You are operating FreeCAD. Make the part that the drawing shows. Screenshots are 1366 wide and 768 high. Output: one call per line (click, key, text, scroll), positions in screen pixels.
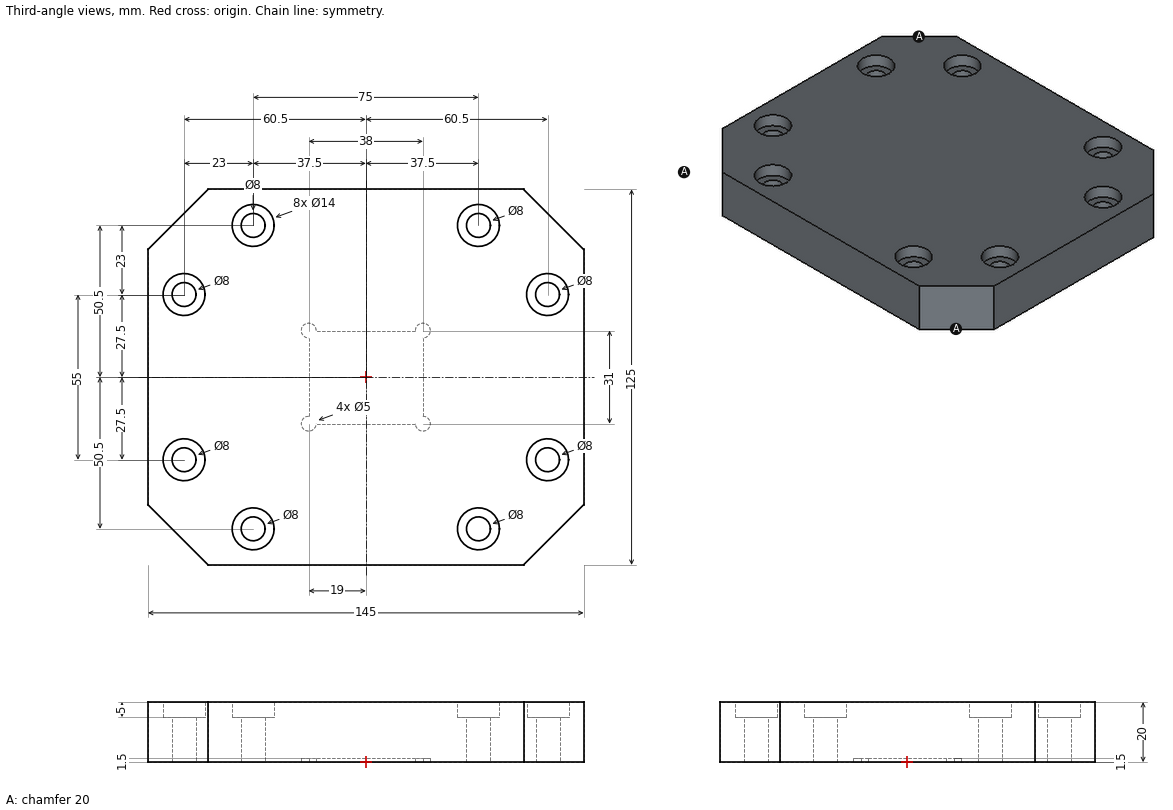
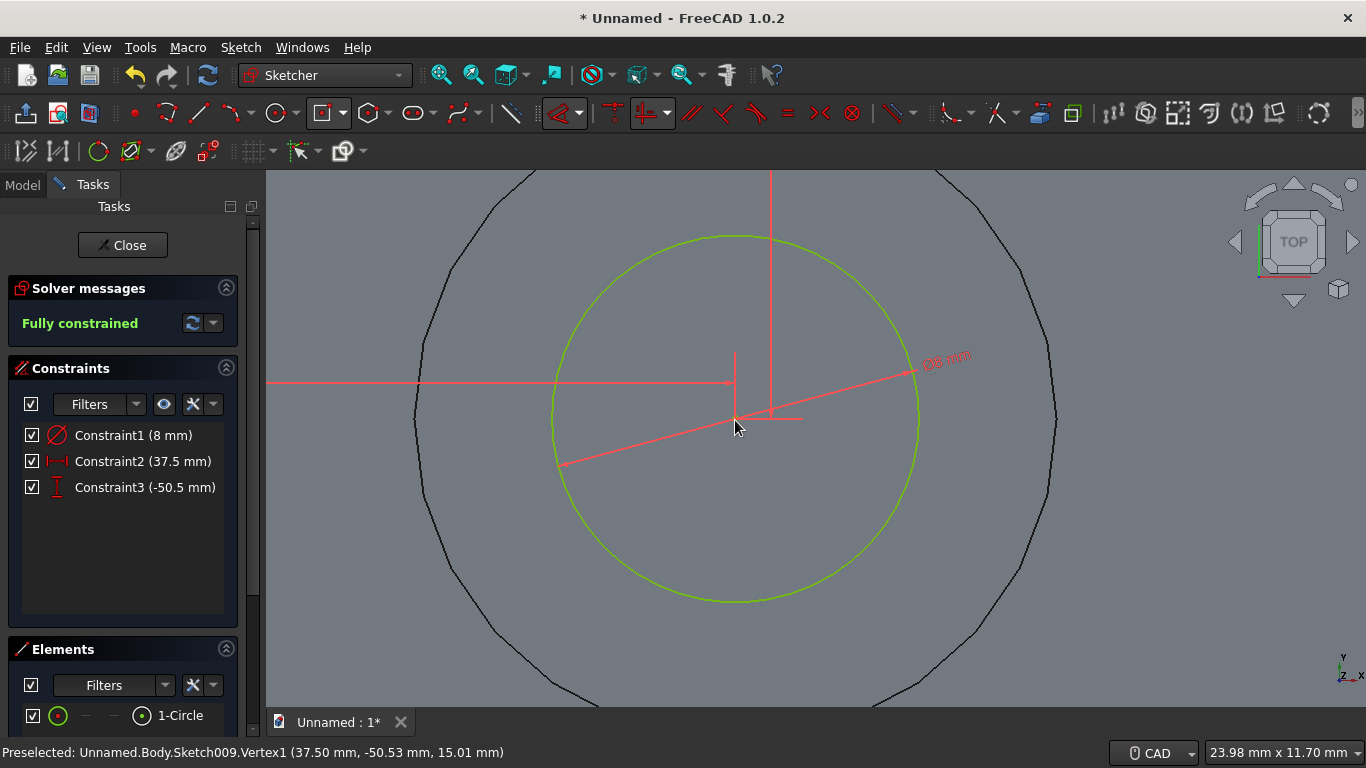
click(123, 245)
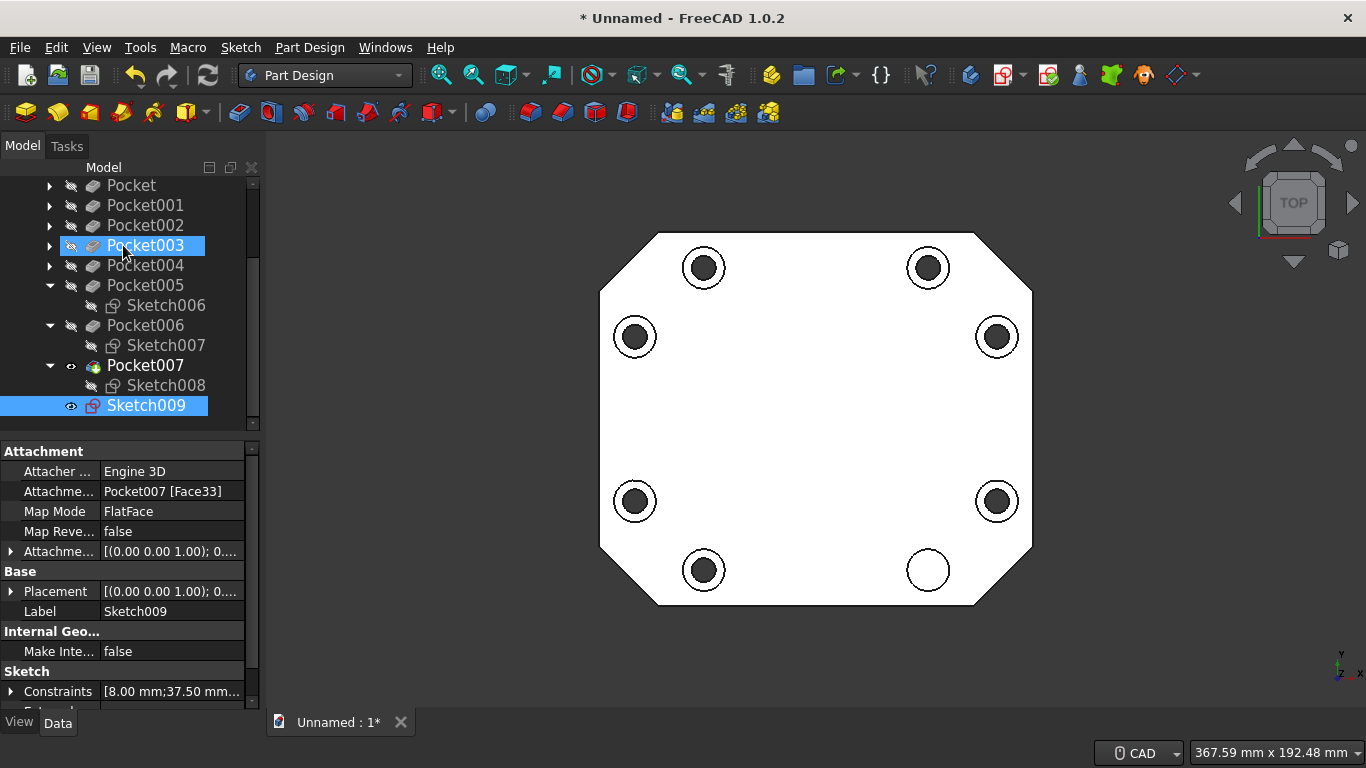
click(240, 112)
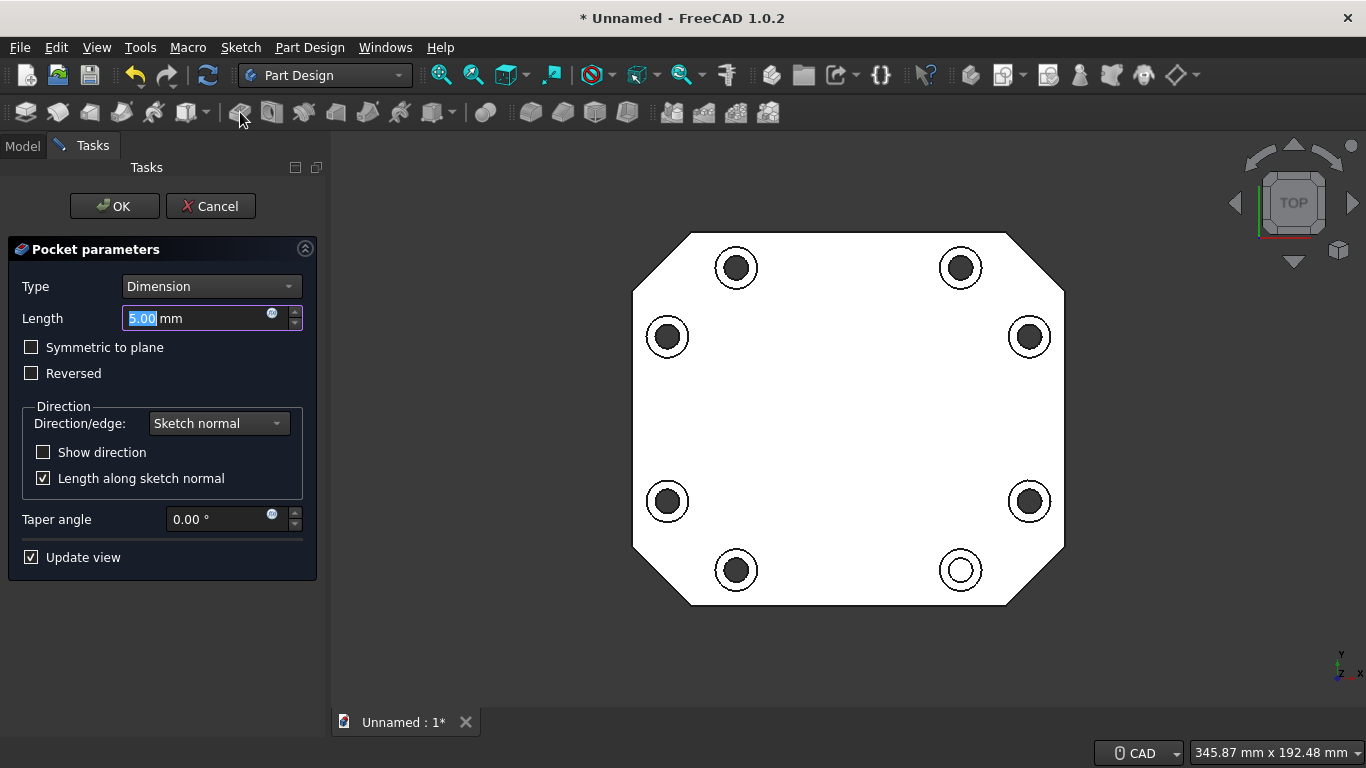
click(212, 286)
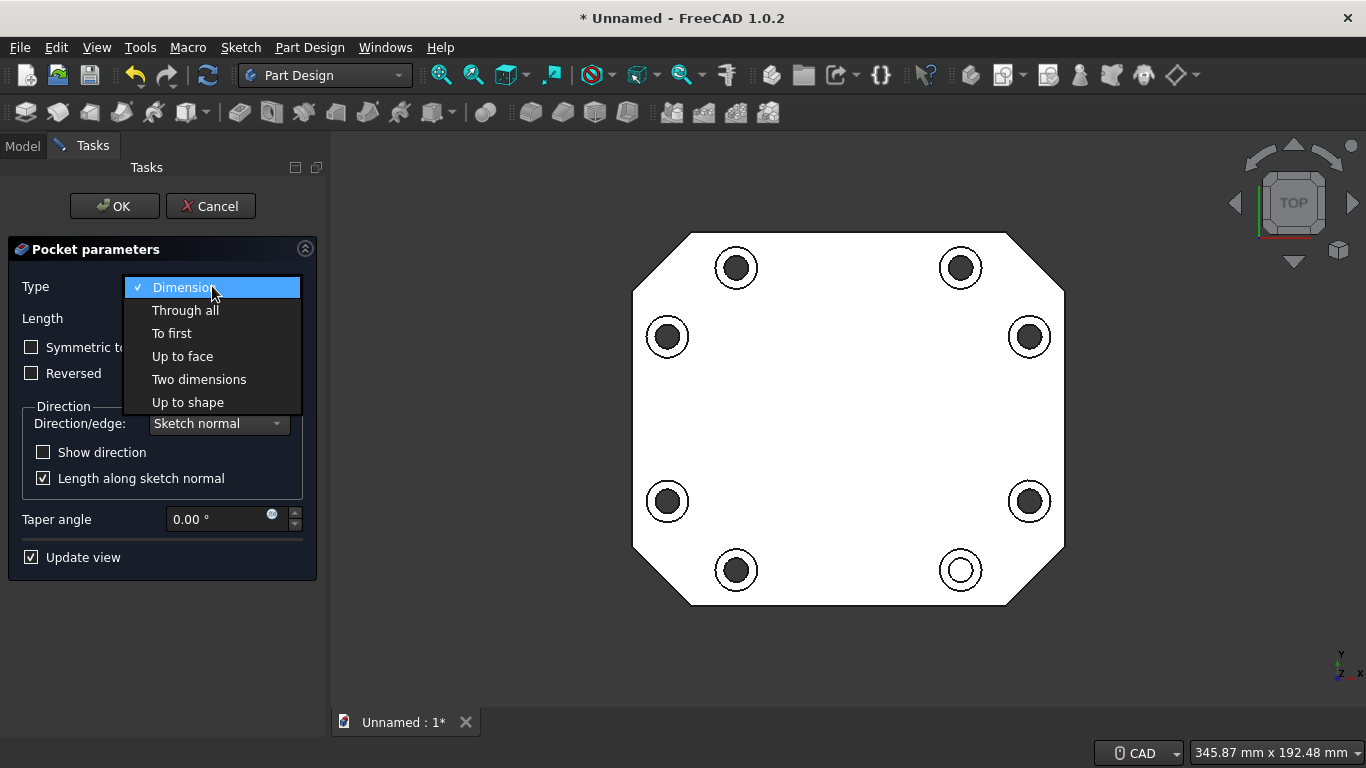
click(212, 334)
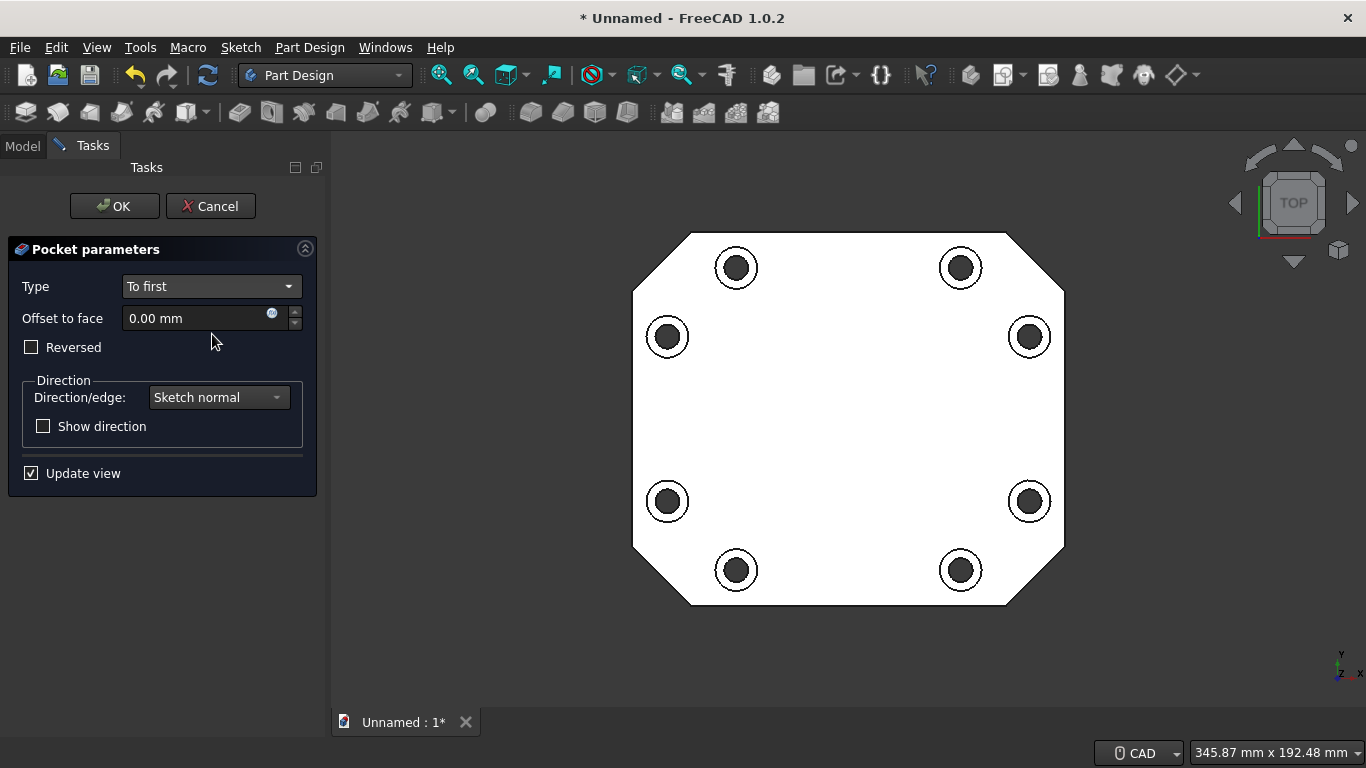
click(115, 206)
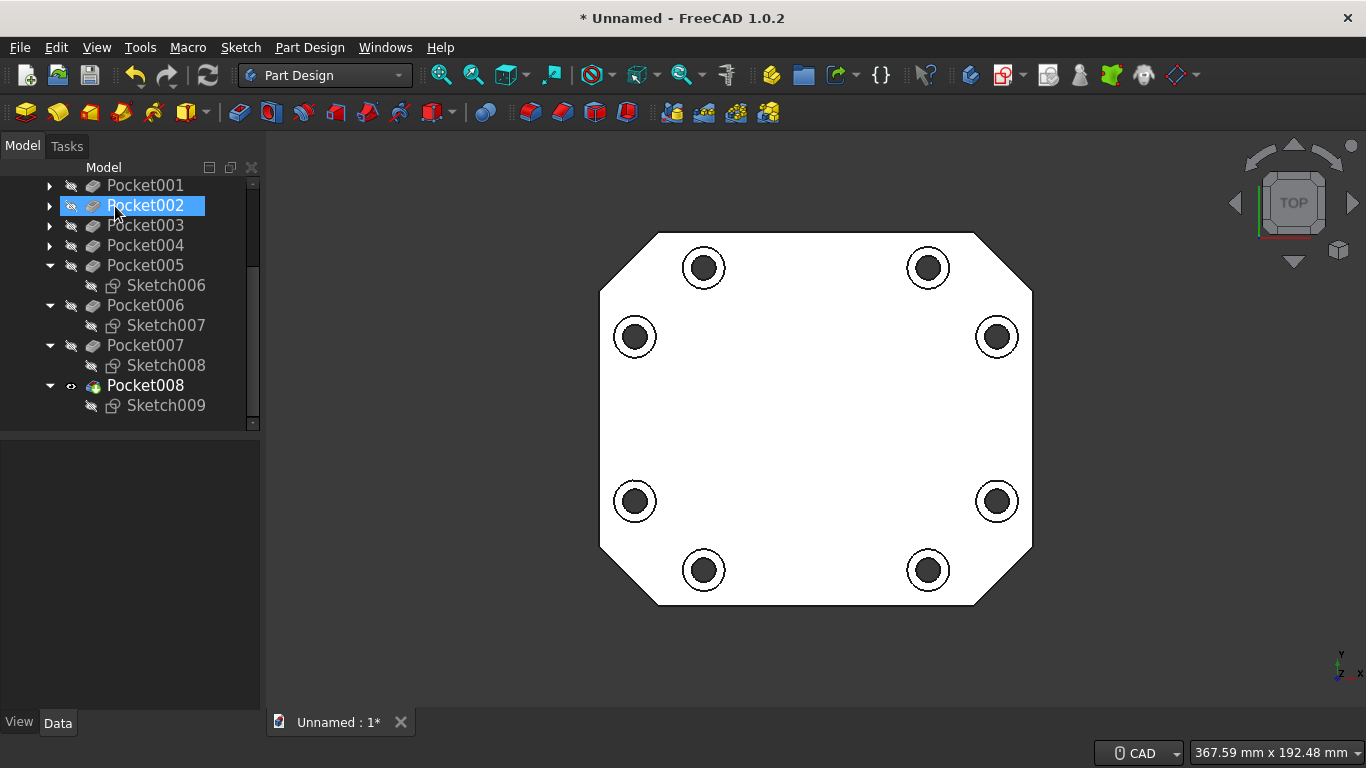
key(5)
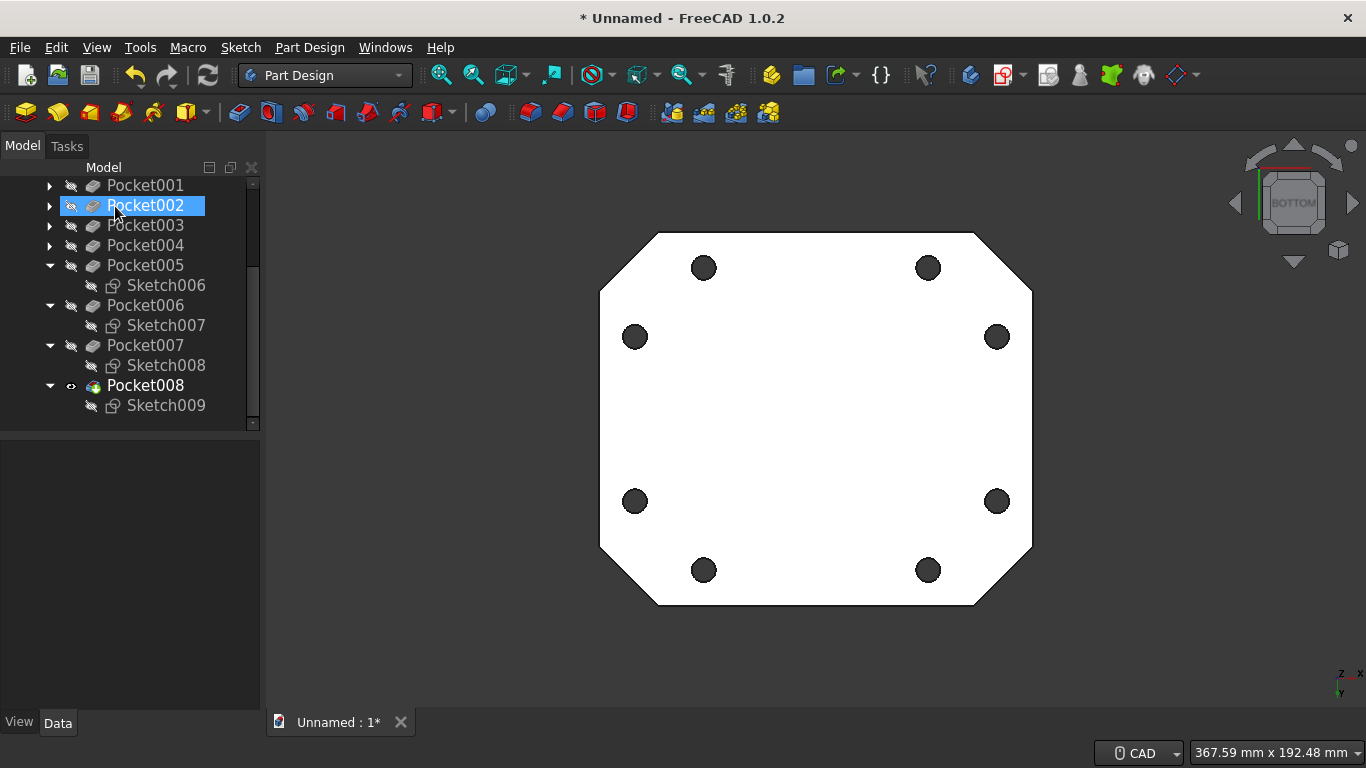
click(816, 418)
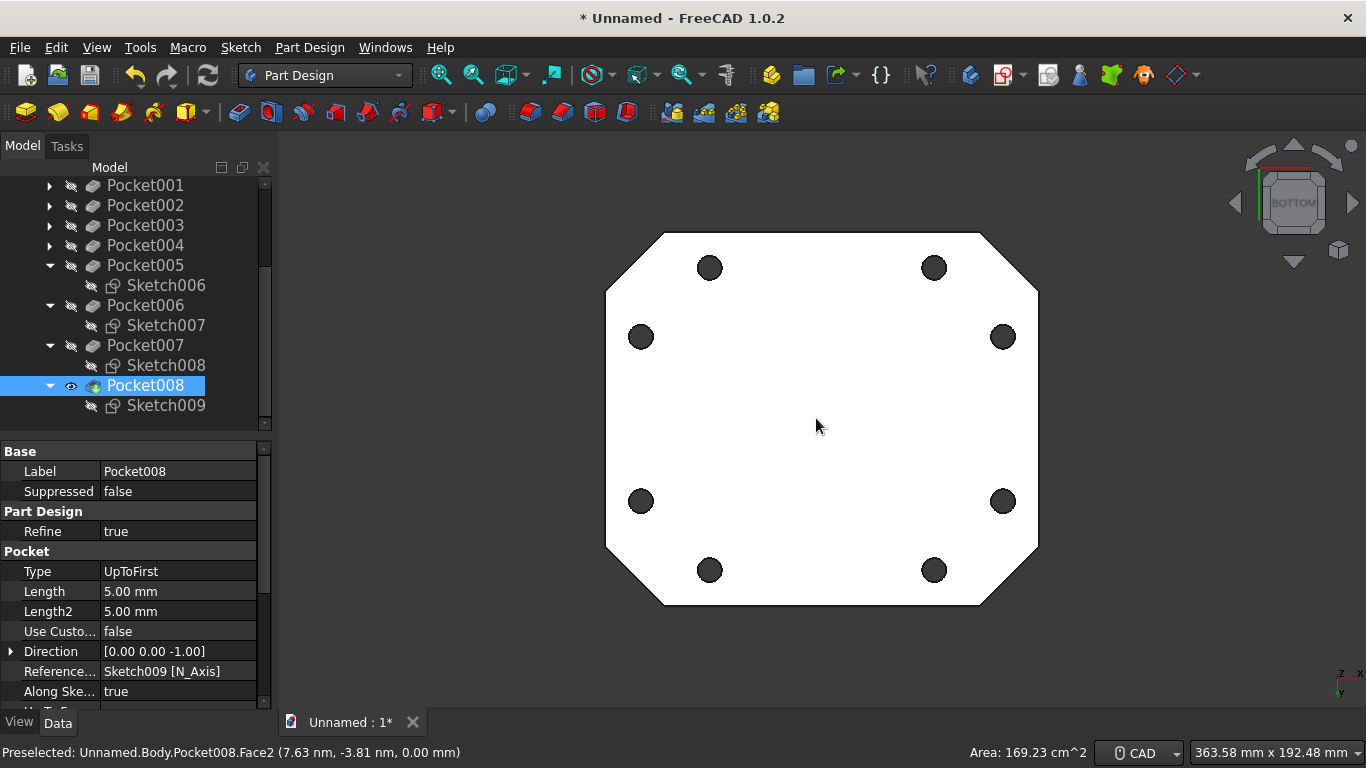
click(1004, 76)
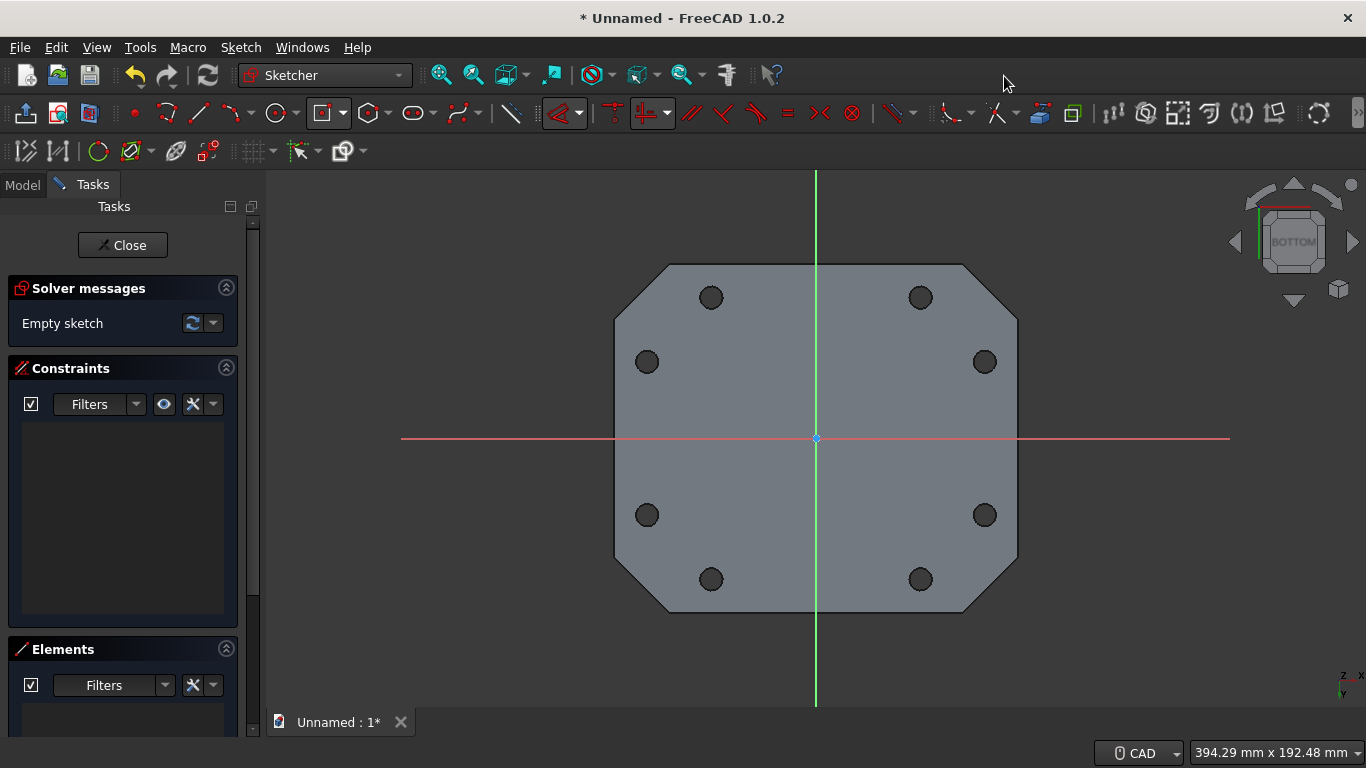
scroll(838, 439, up, 7)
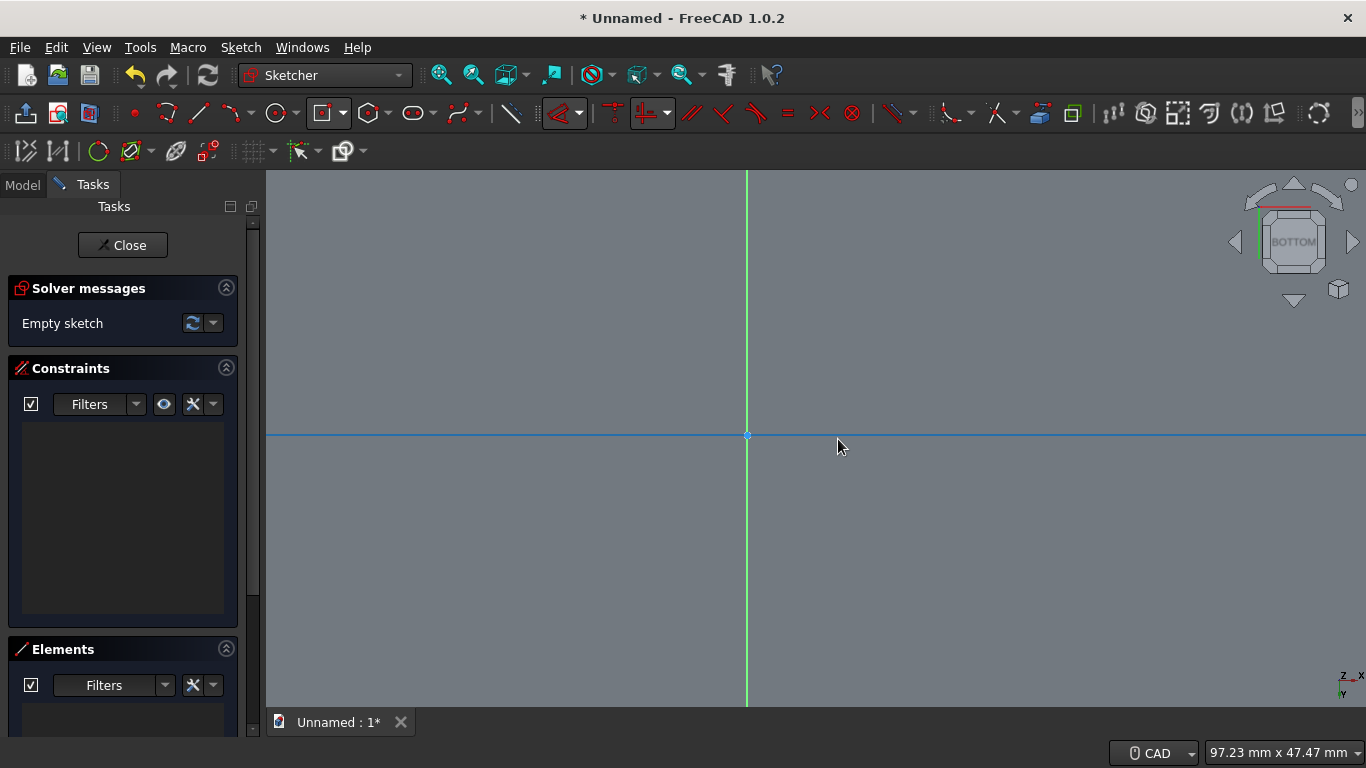
click(322, 114)